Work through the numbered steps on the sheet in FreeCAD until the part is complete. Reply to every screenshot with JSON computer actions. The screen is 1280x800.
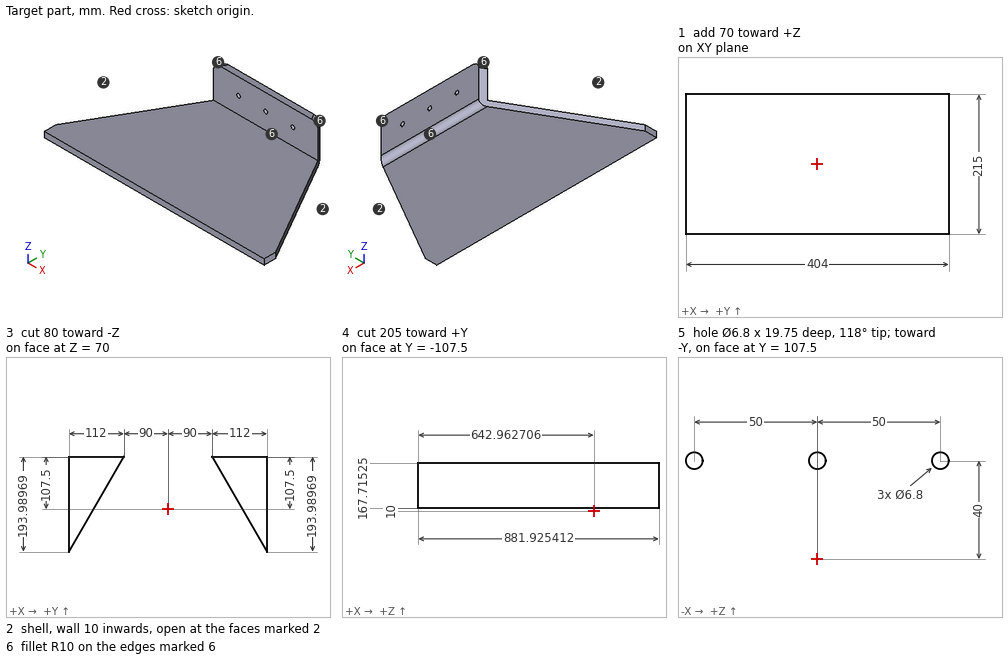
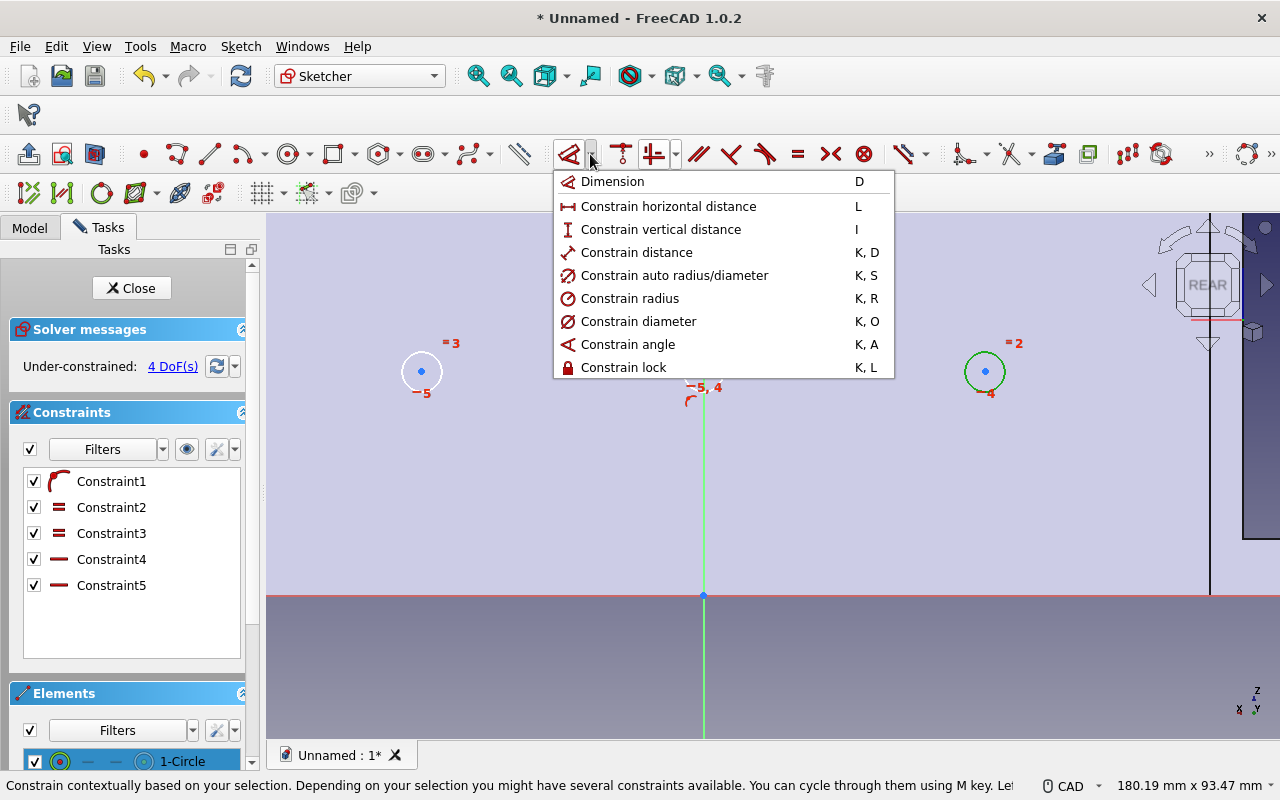
{"action": "left_click", "coordinate": [724, 322]}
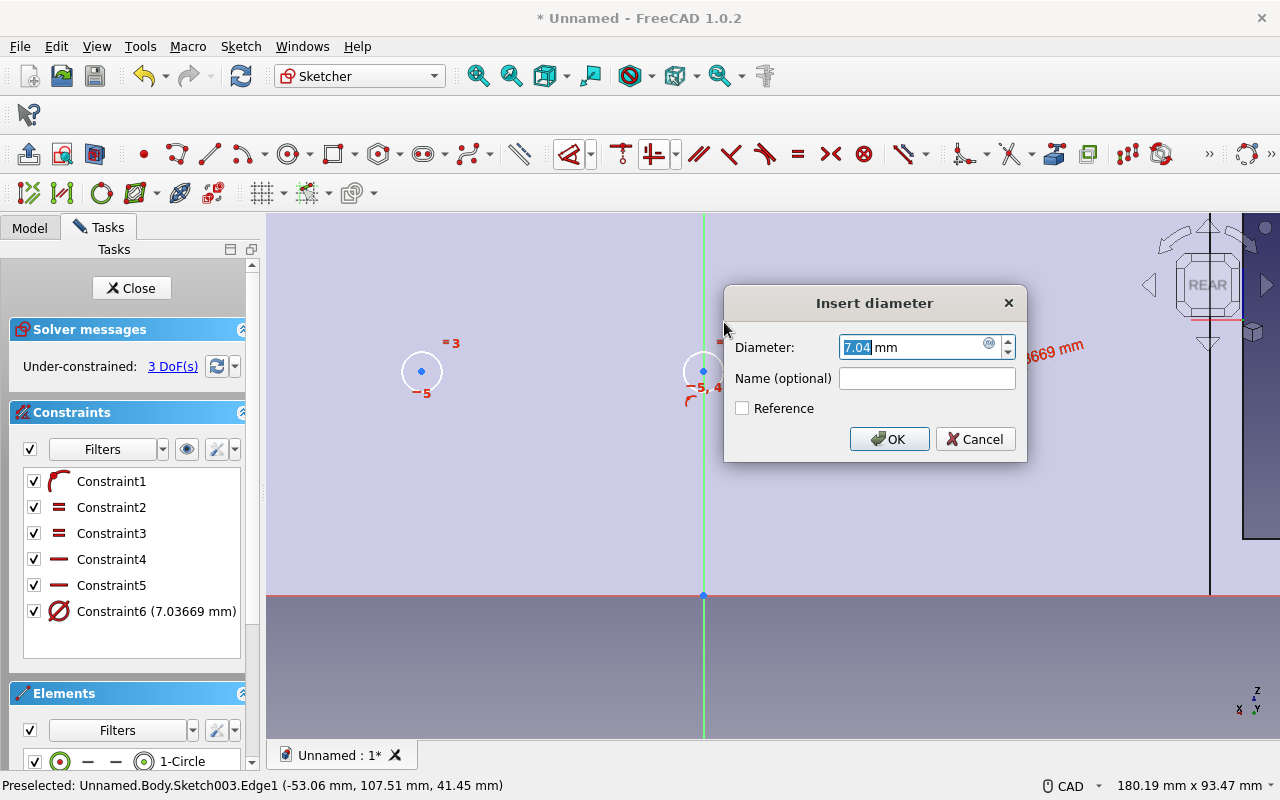
{"action": "type", "text": "6.8"}
{"action": "key", "text": "Return"}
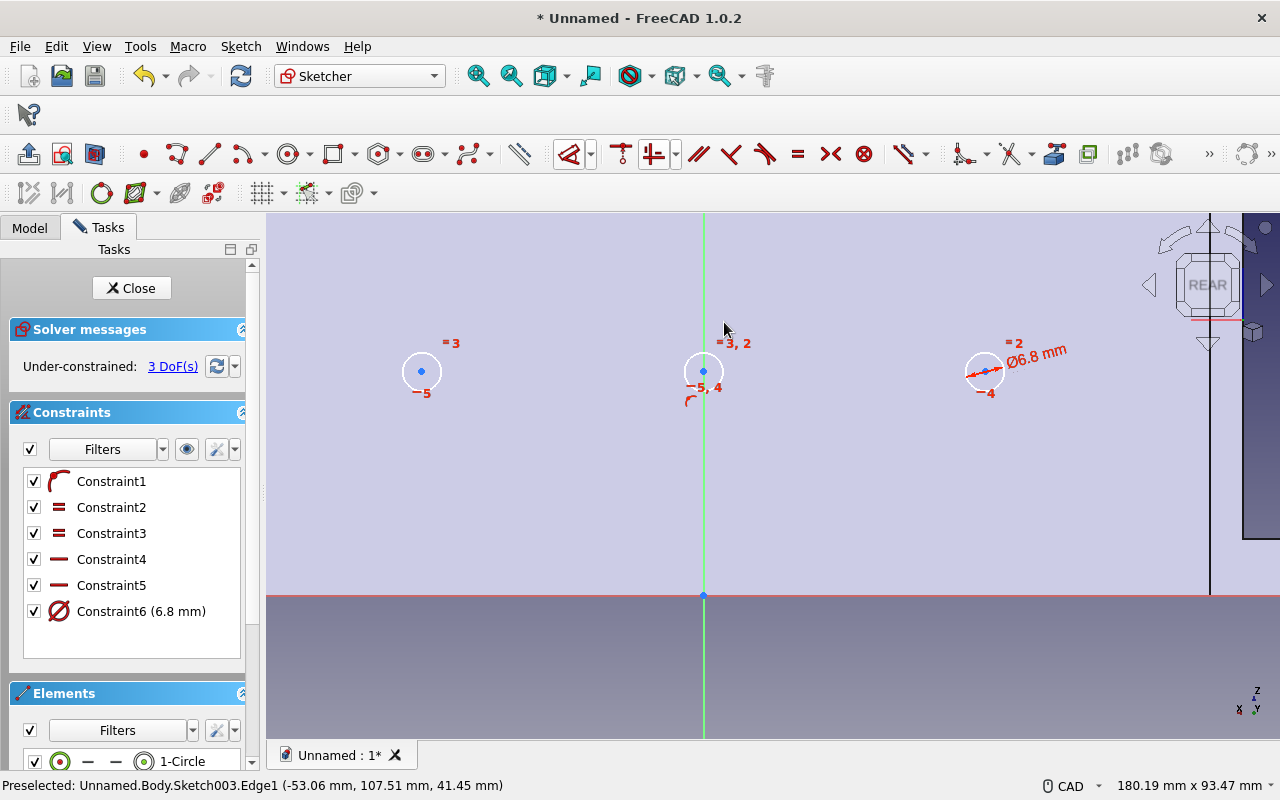
{"action": "left_click", "coordinate": [985, 372]}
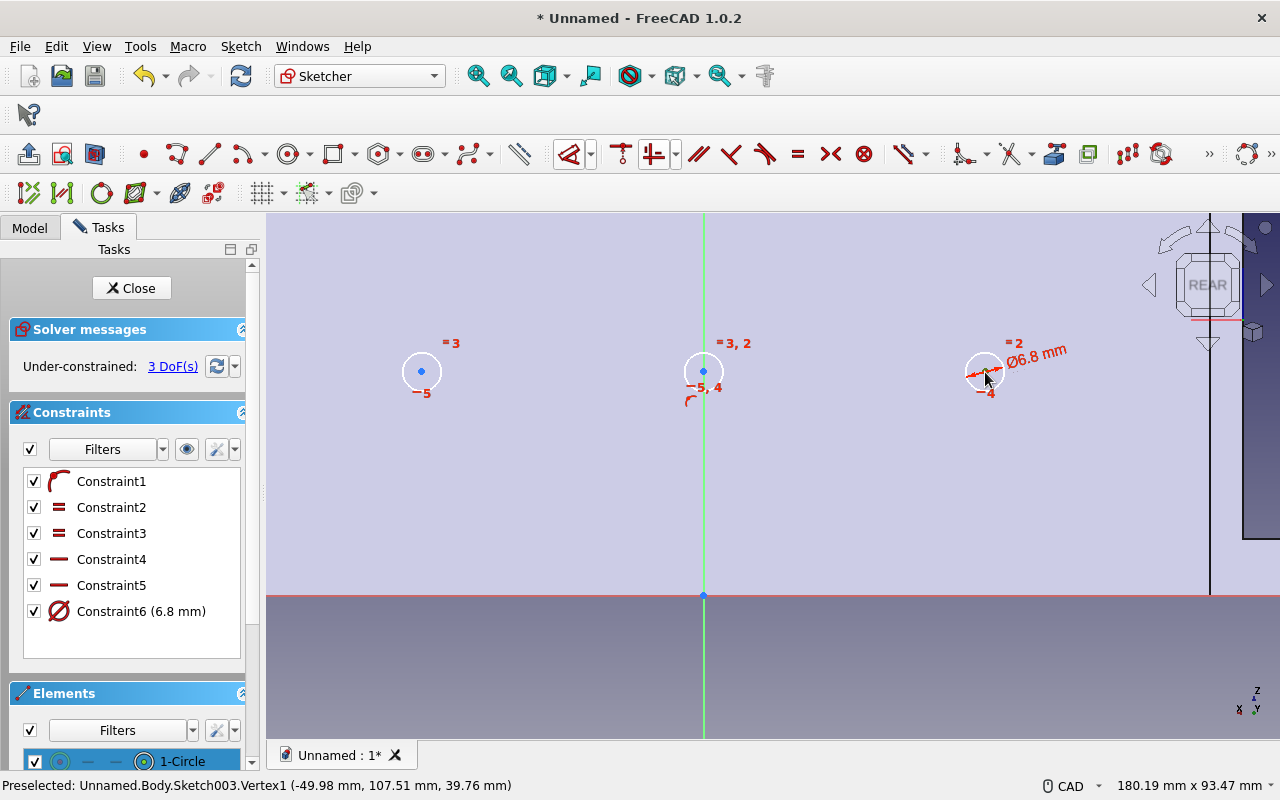
{"action": "key", "text": "l"}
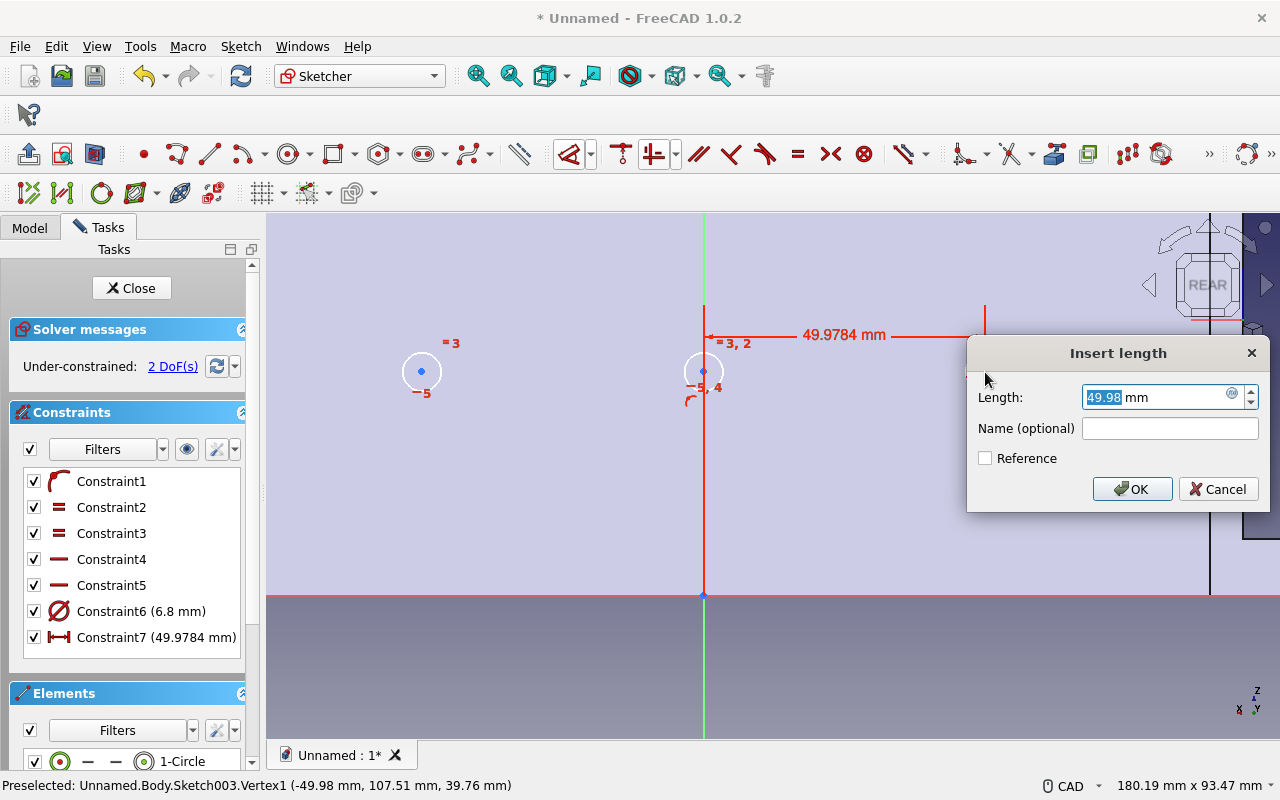
{"action": "type", "text": "50"}
{"action": "key", "text": "Return"}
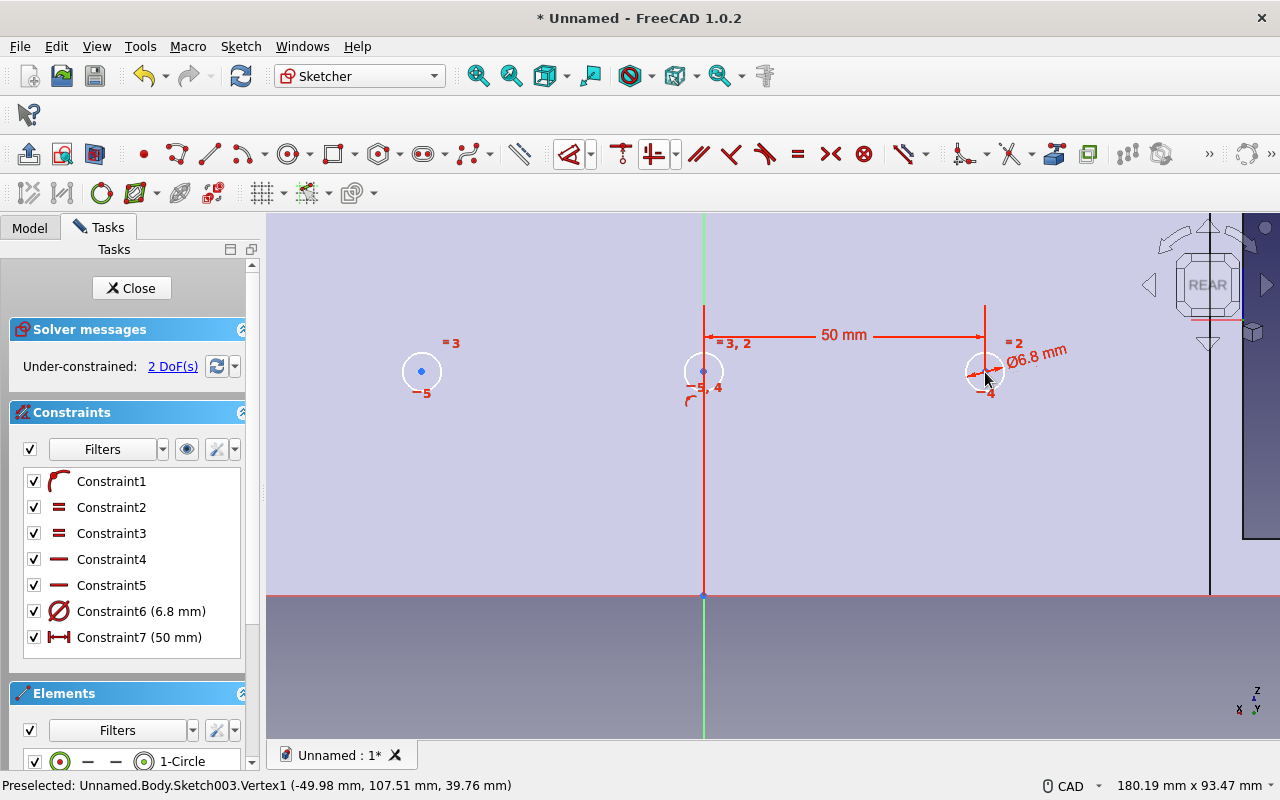
{"action": "left_click", "coordinate": [985, 372]}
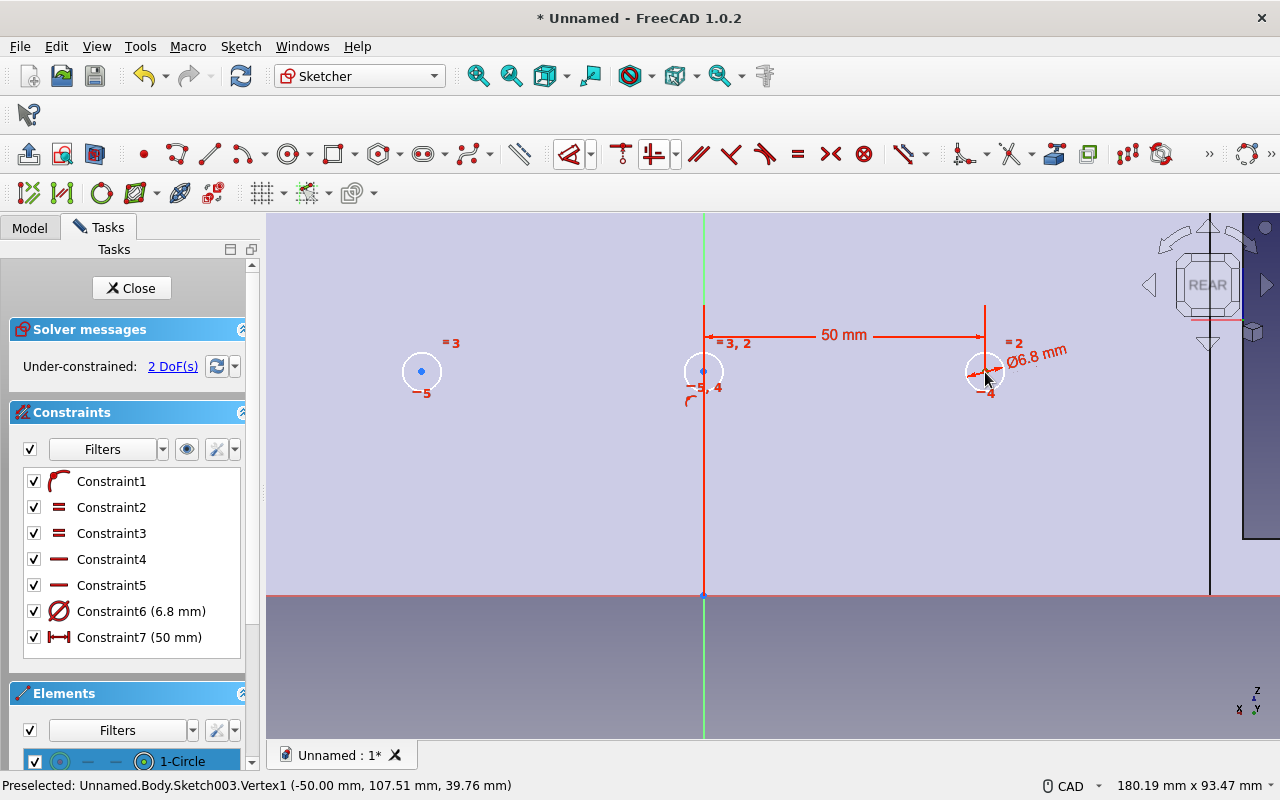
{"action": "left_click", "coordinate": [590, 154]}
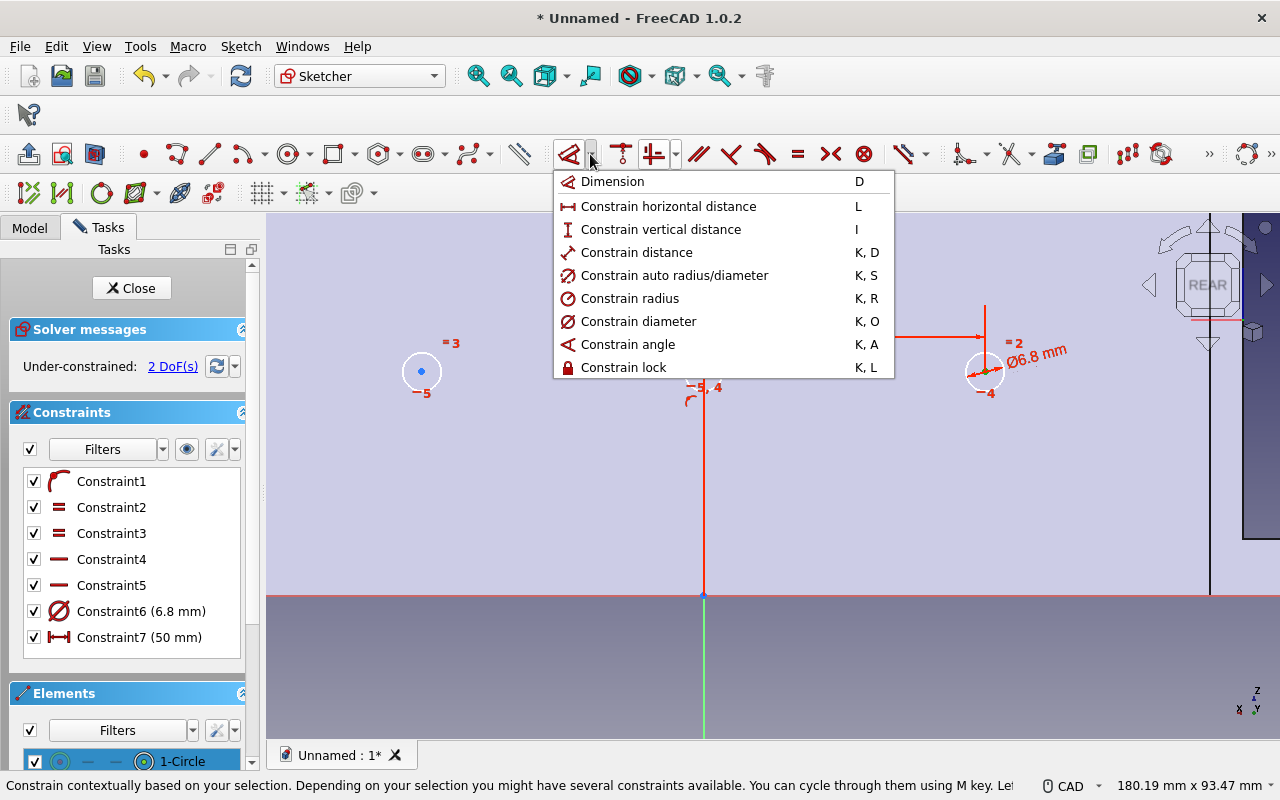
{"action": "left_click", "coordinate": [724, 230]}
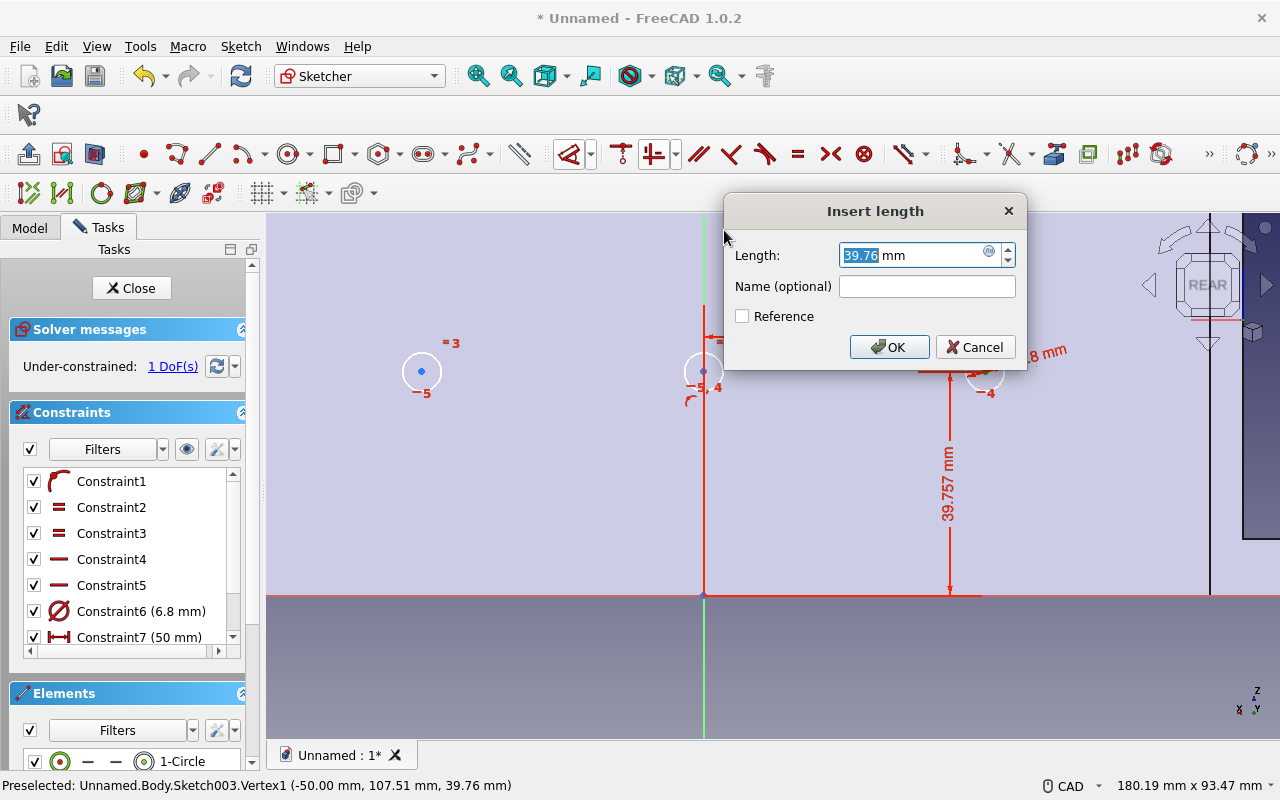
{"action": "type", "text": "40"}
{"action": "key", "text": "Return"}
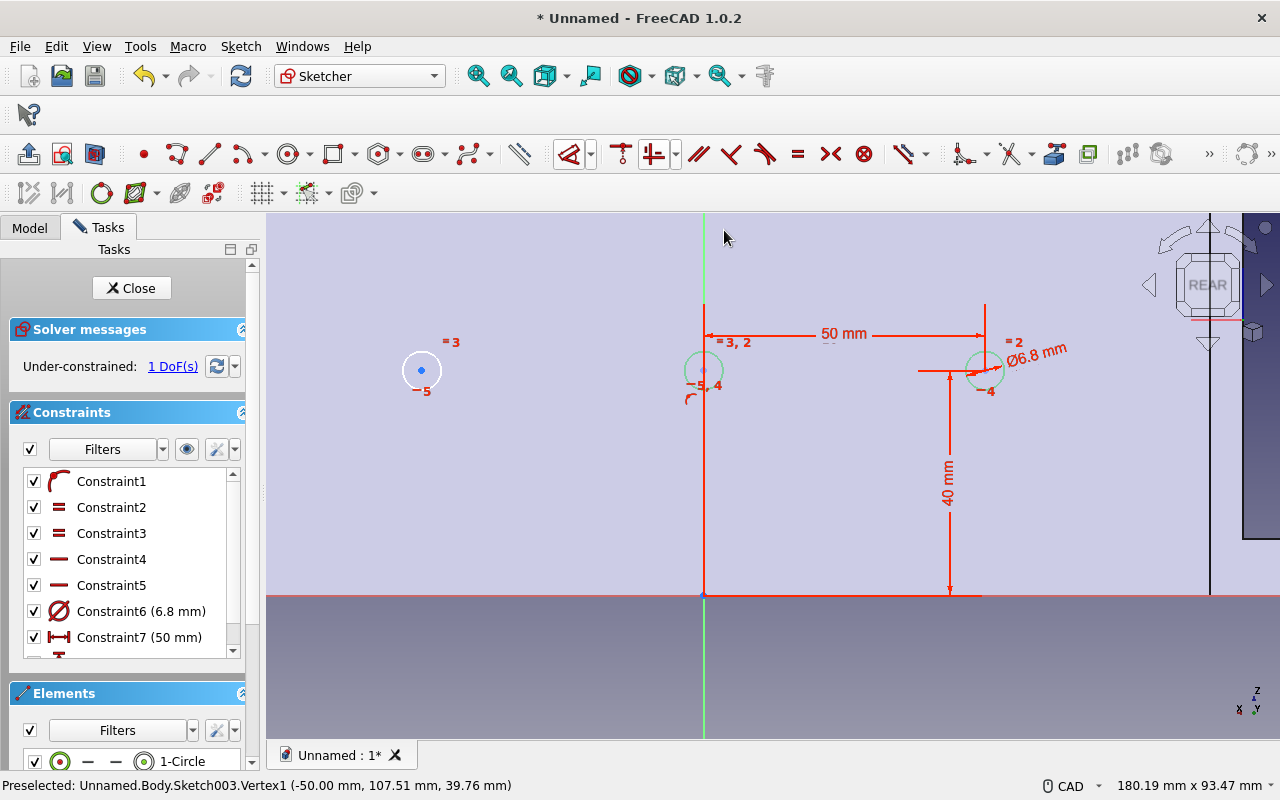
{"action": "left_click", "coordinate": [422, 371]}